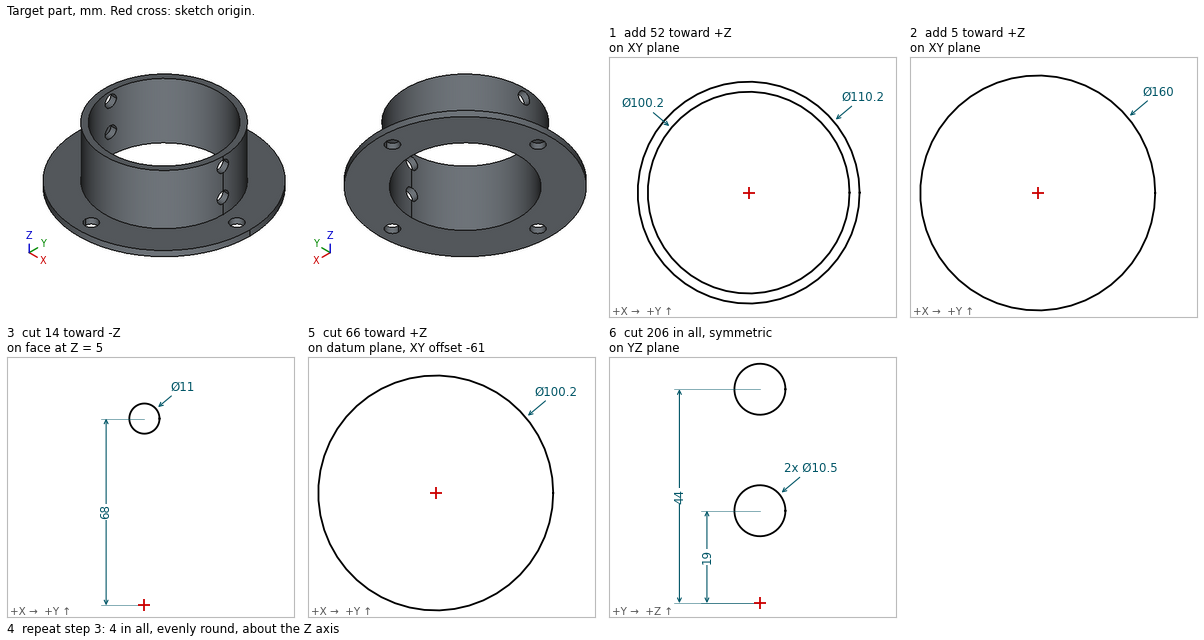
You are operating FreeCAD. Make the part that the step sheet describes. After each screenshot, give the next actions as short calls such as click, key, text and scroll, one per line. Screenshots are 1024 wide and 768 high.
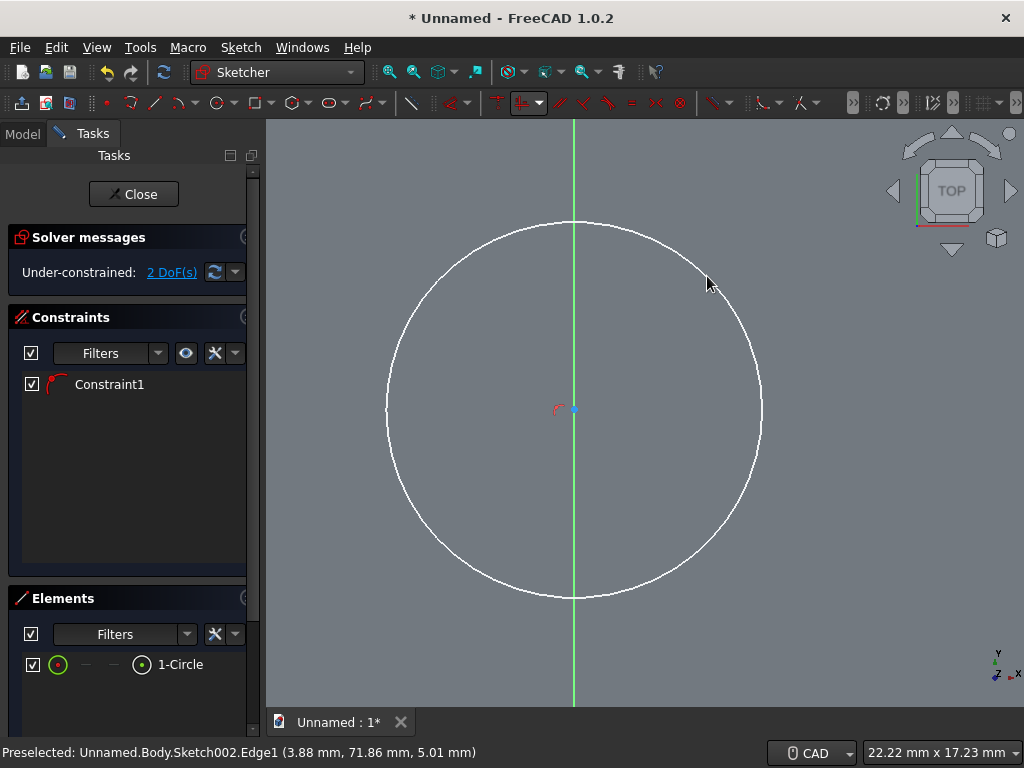
click(450, 104)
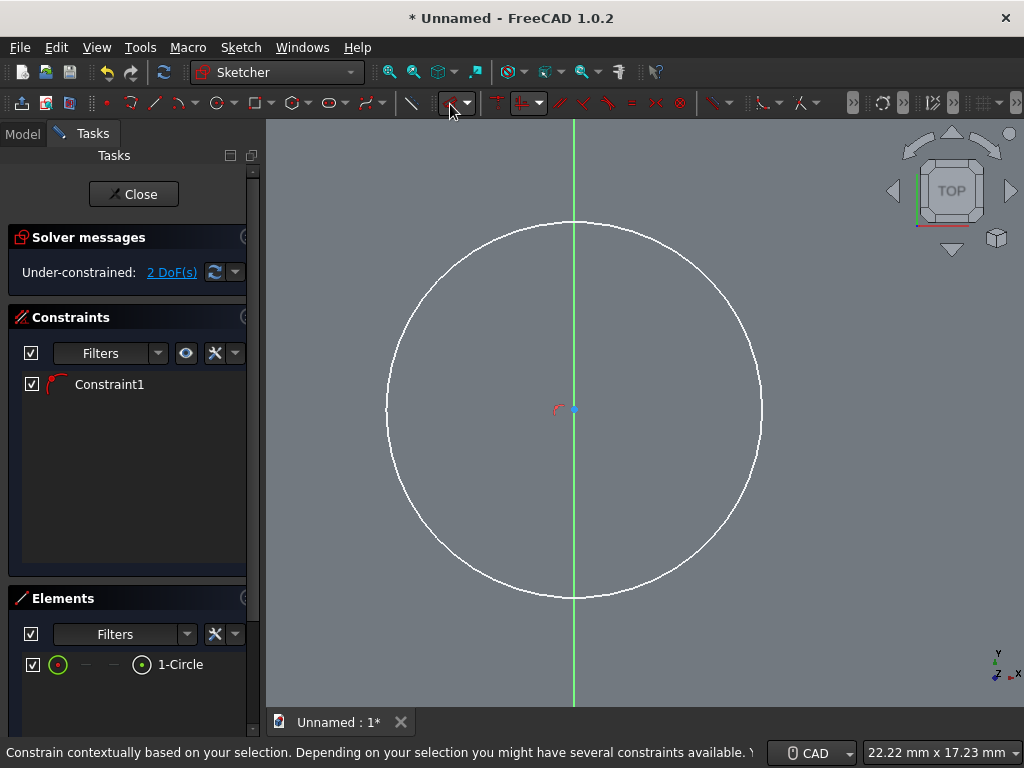
click(707, 277)
click(730, 254)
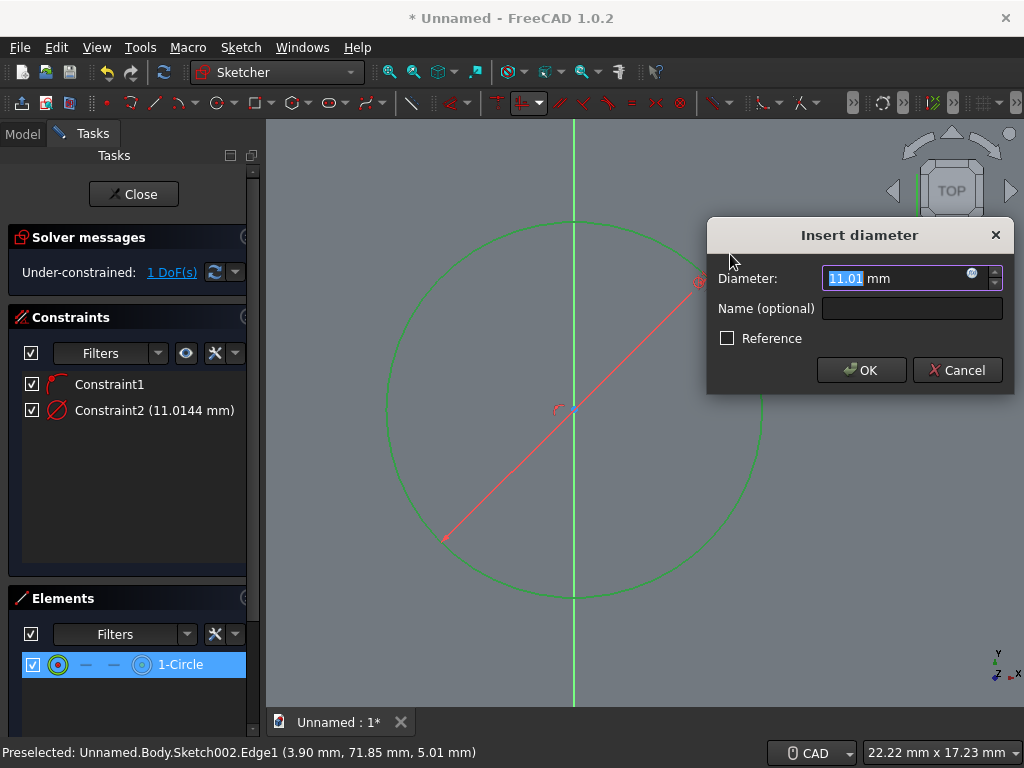
text(11)
key(Return)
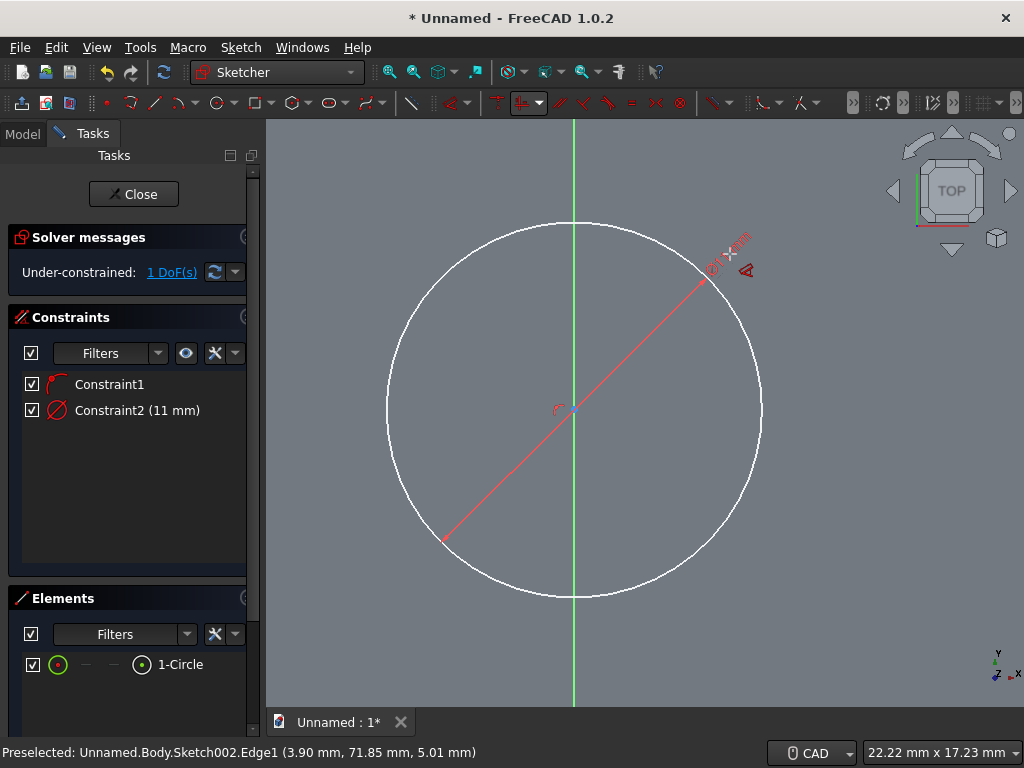
click(574, 410)
click(608, 544)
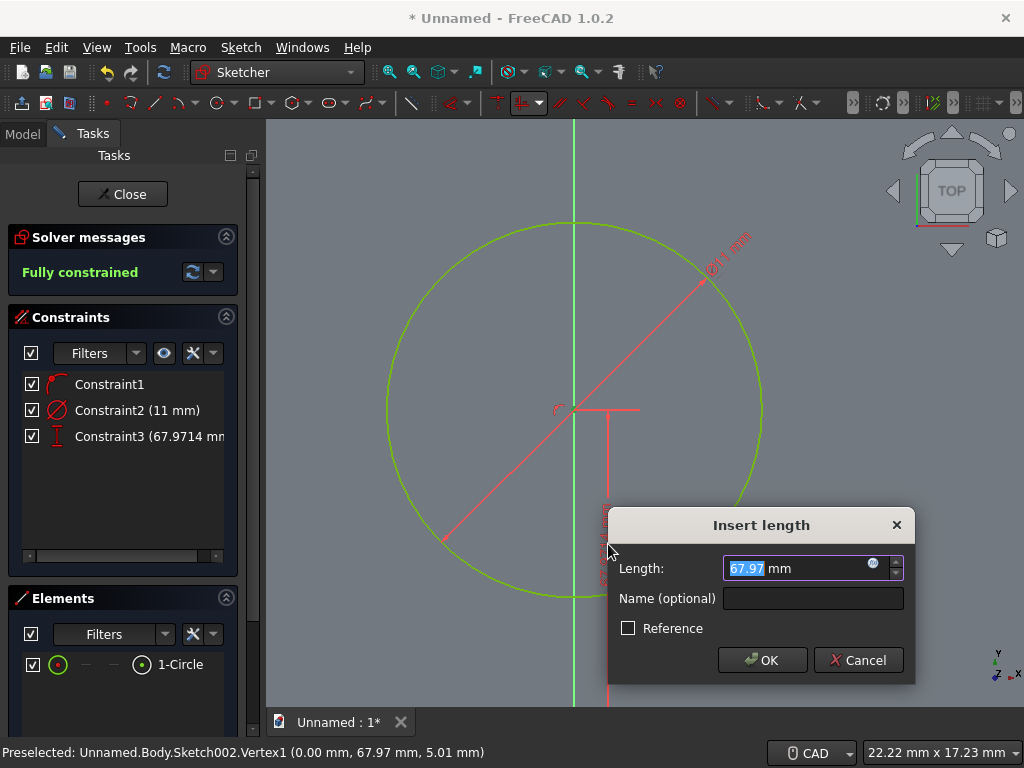
text(68)
key(Return)
key(Escape)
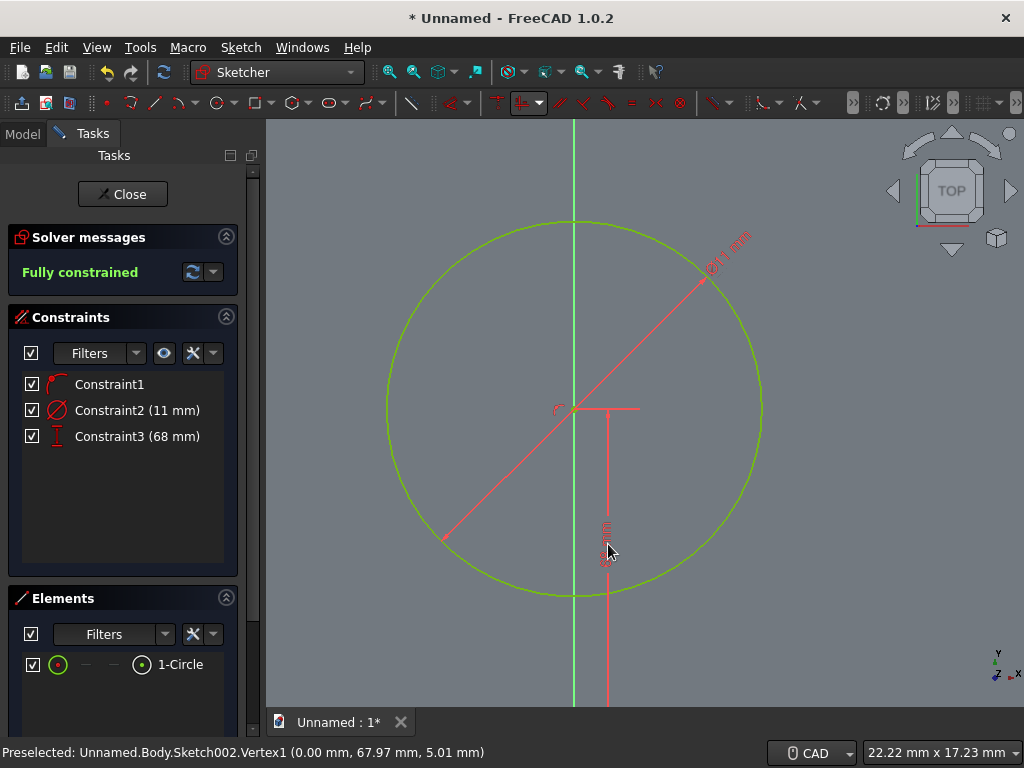
click(123, 194)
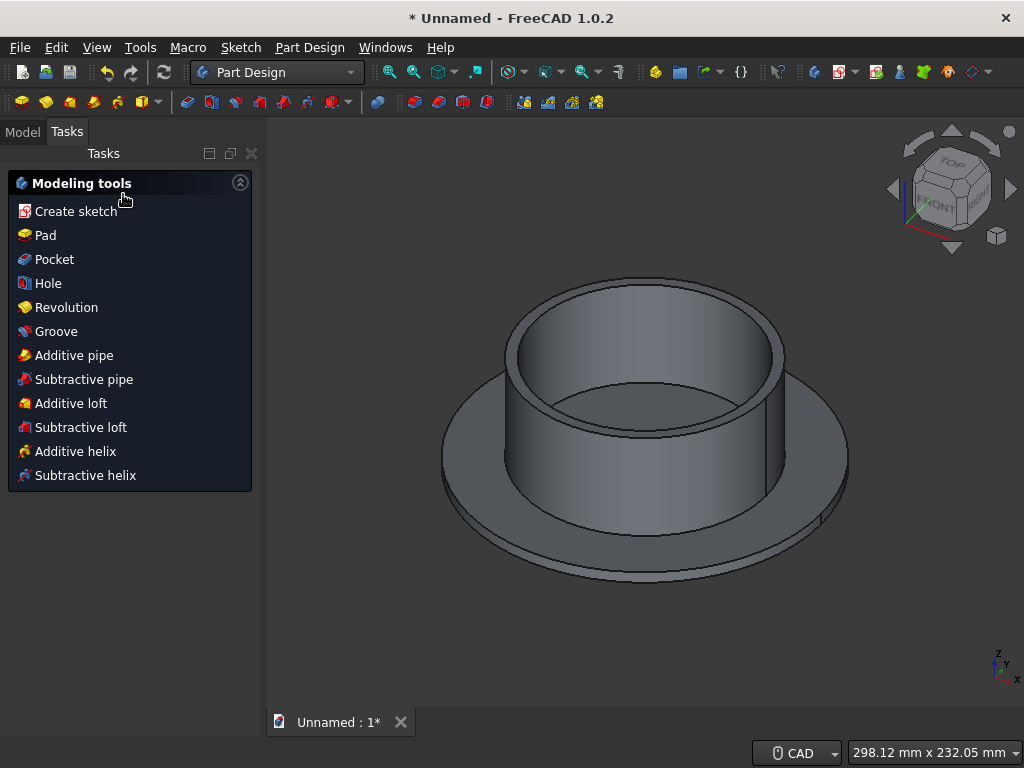
click(188, 102)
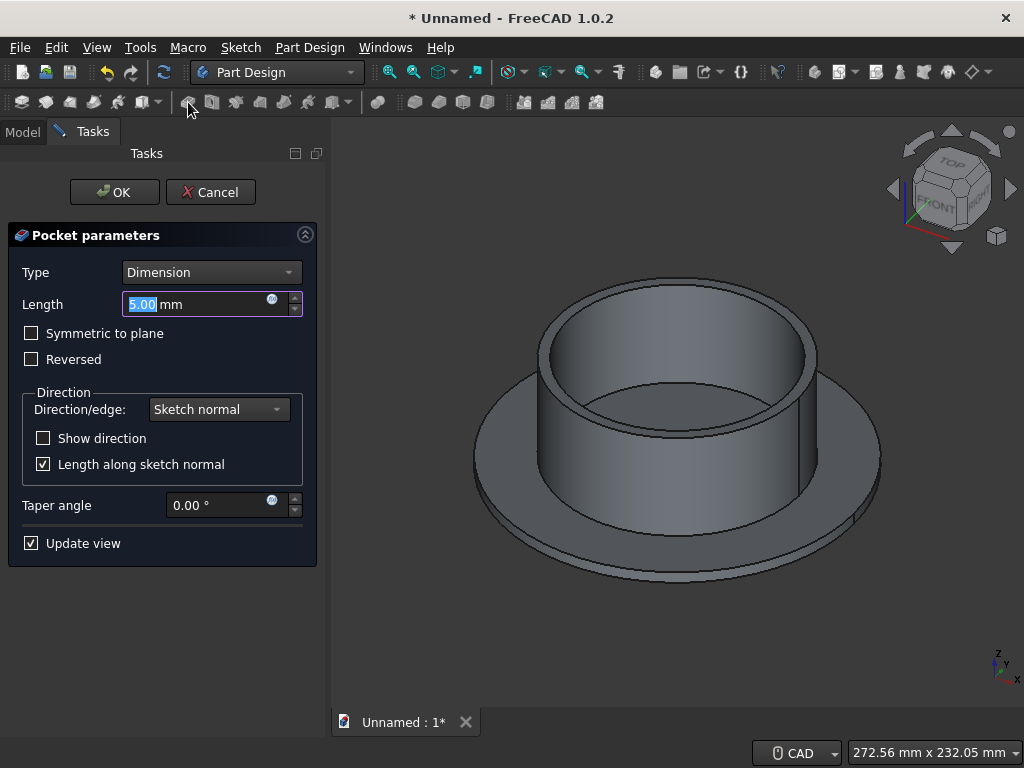
text(14)
key(Tab)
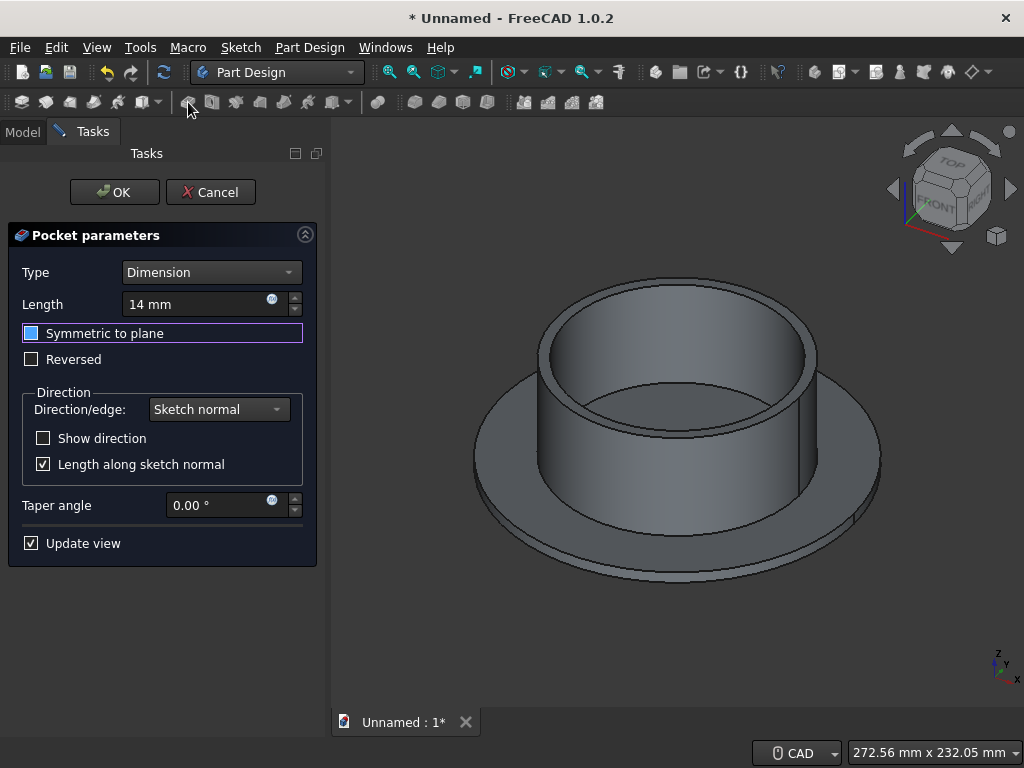
click(115, 192)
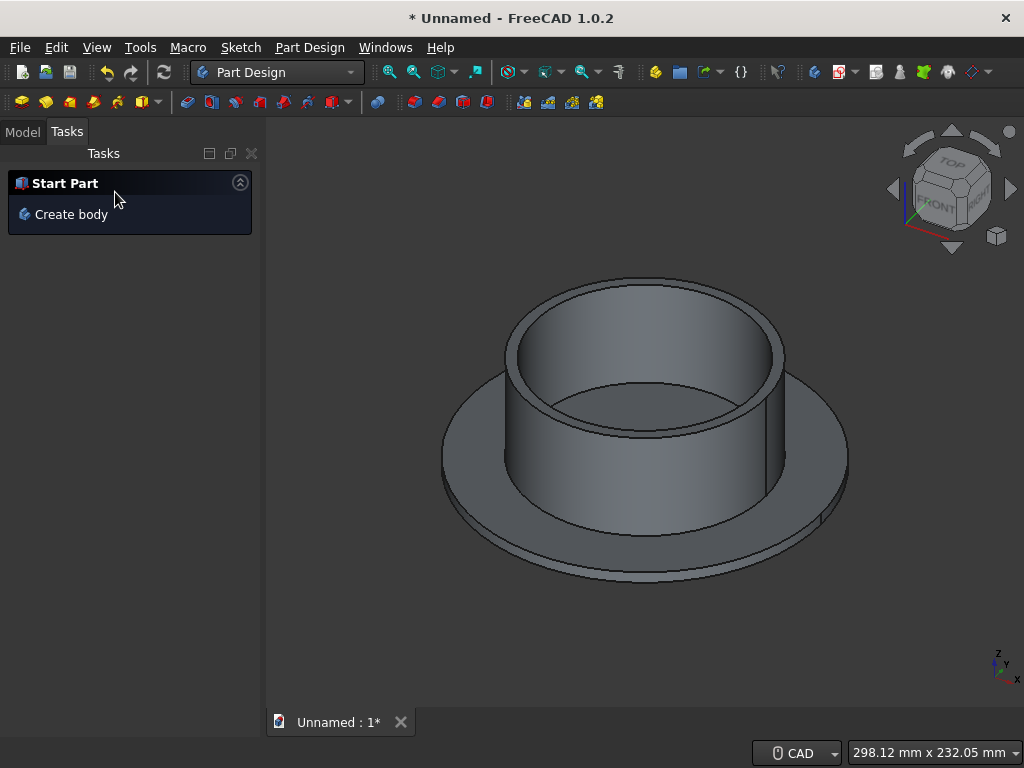
click(23, 131)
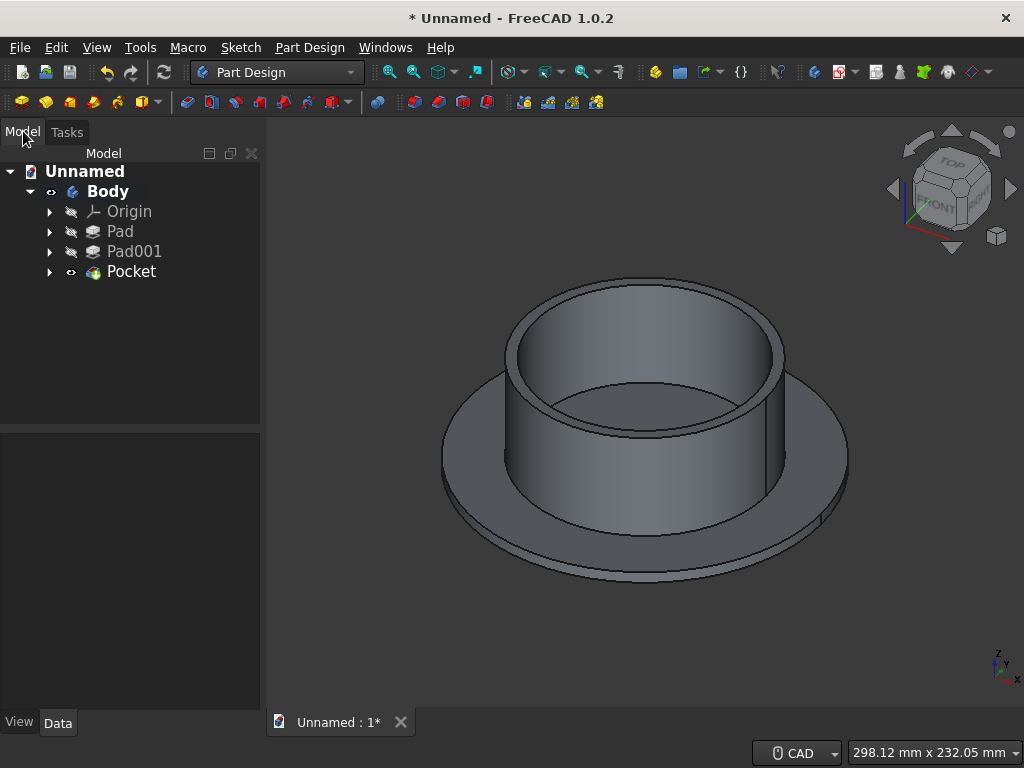
click(116, 272)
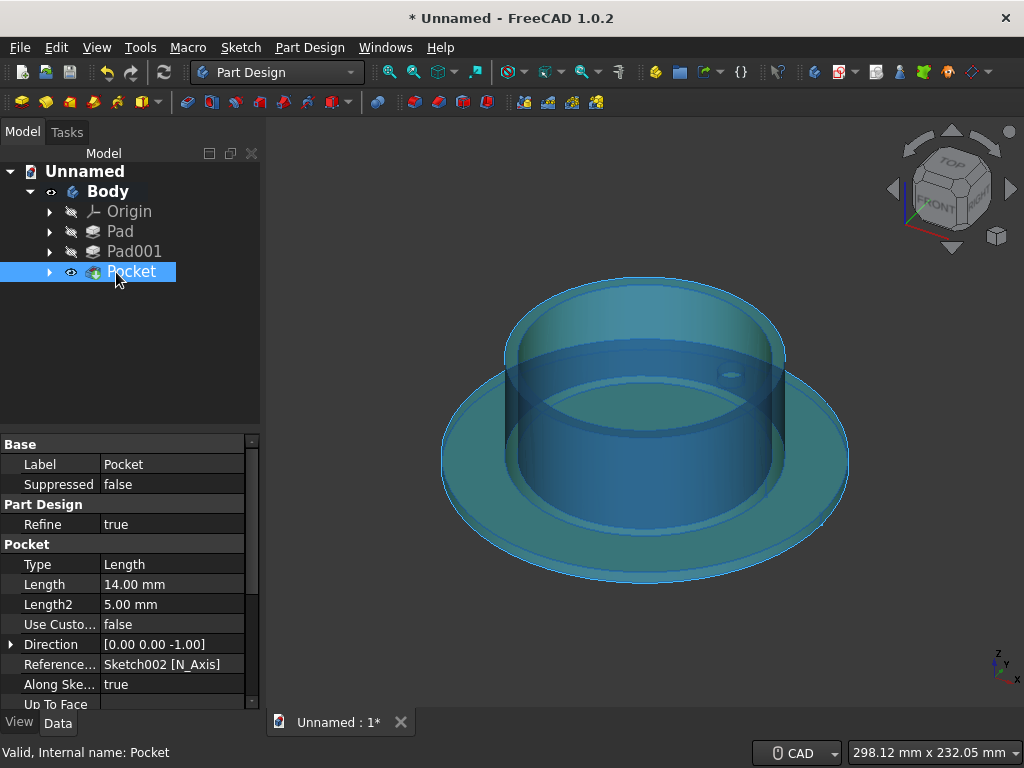
click(572, 102)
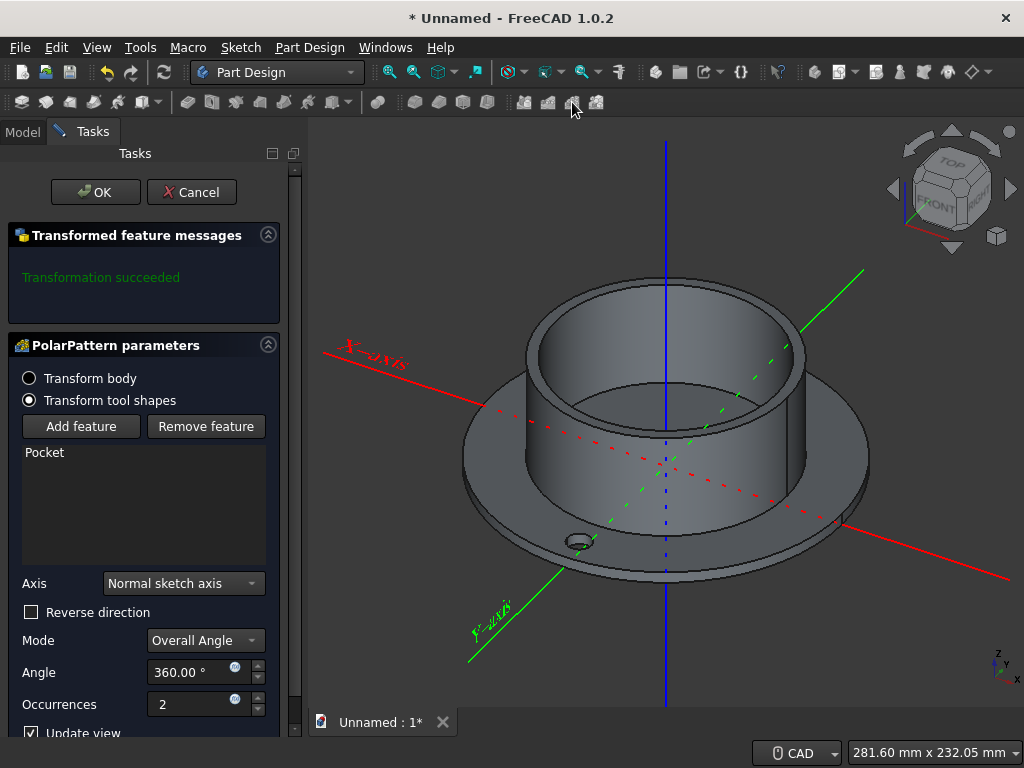
click(184, 584)